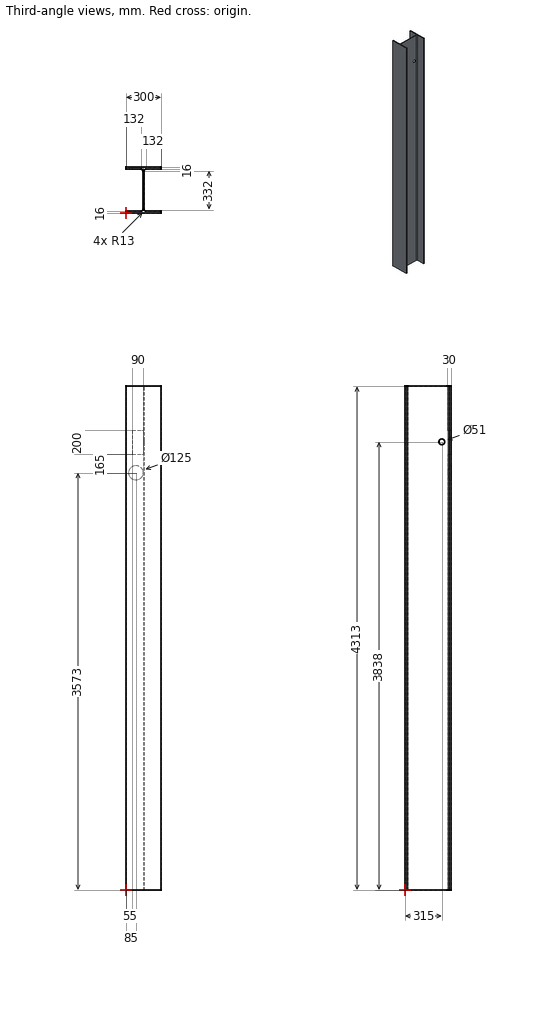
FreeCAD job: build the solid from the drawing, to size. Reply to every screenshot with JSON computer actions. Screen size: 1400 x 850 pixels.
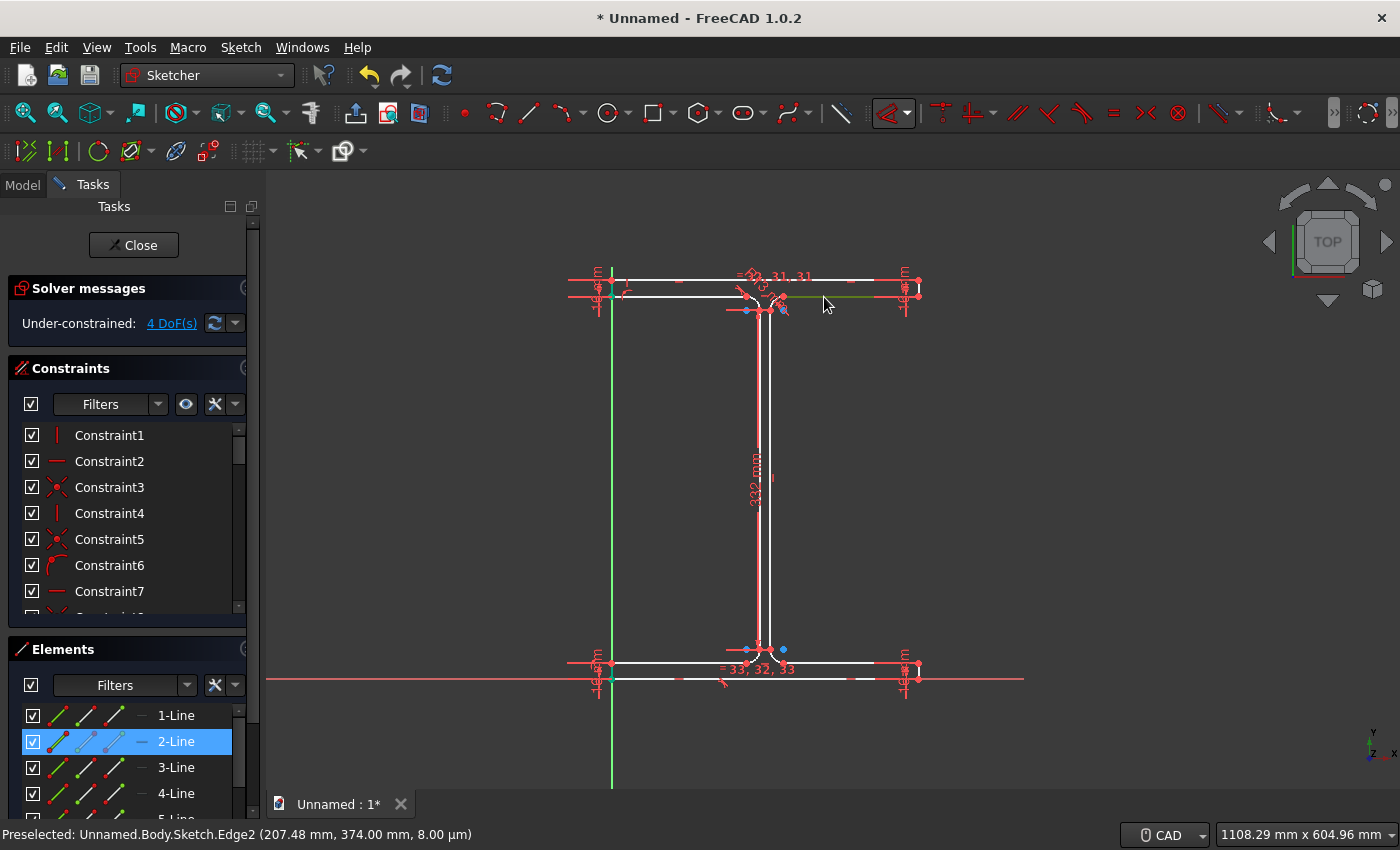
{"action": "left_click", "coordinate": [910, 114]}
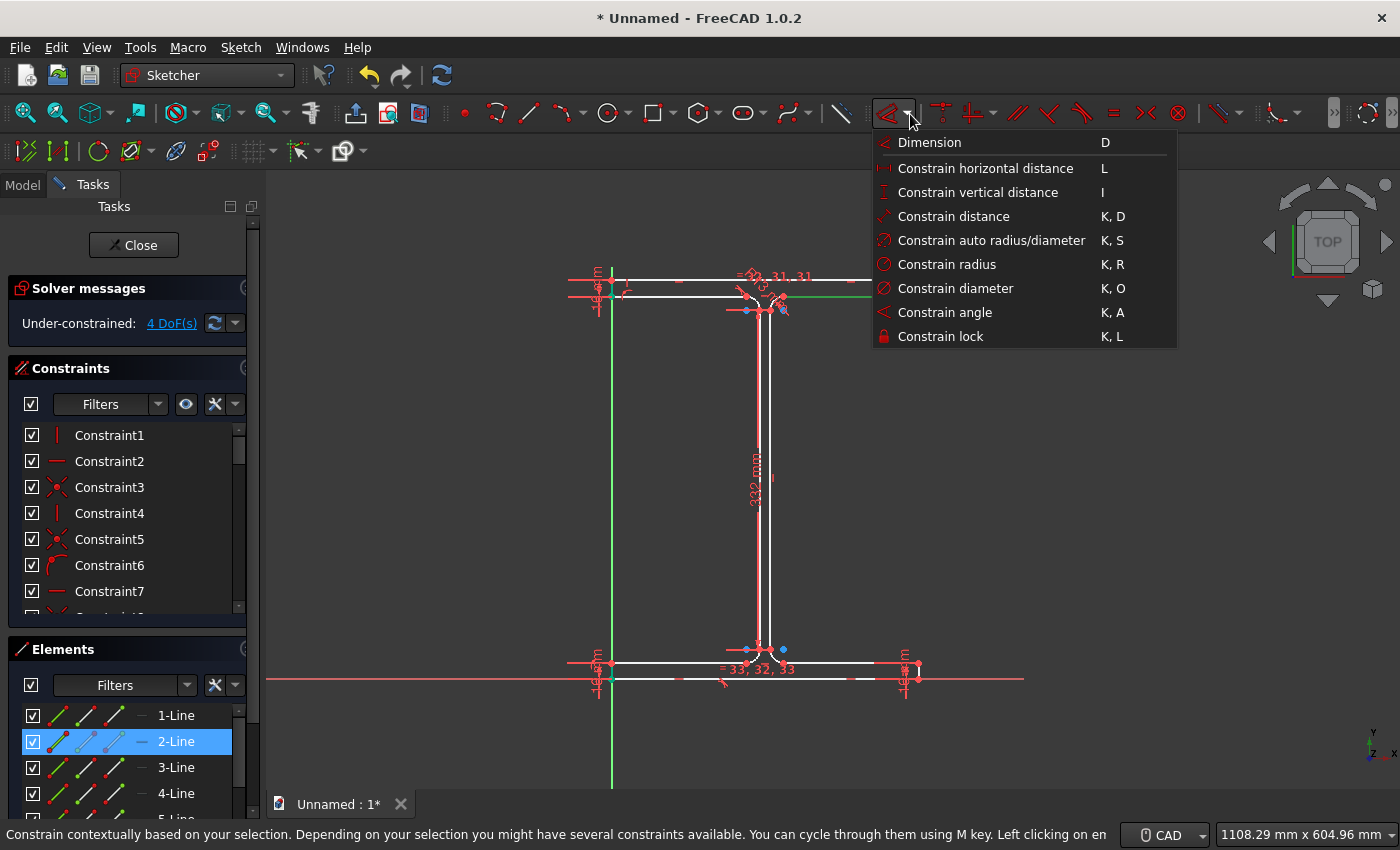
{"action": "left_click", "coordinate": [1025, 168]}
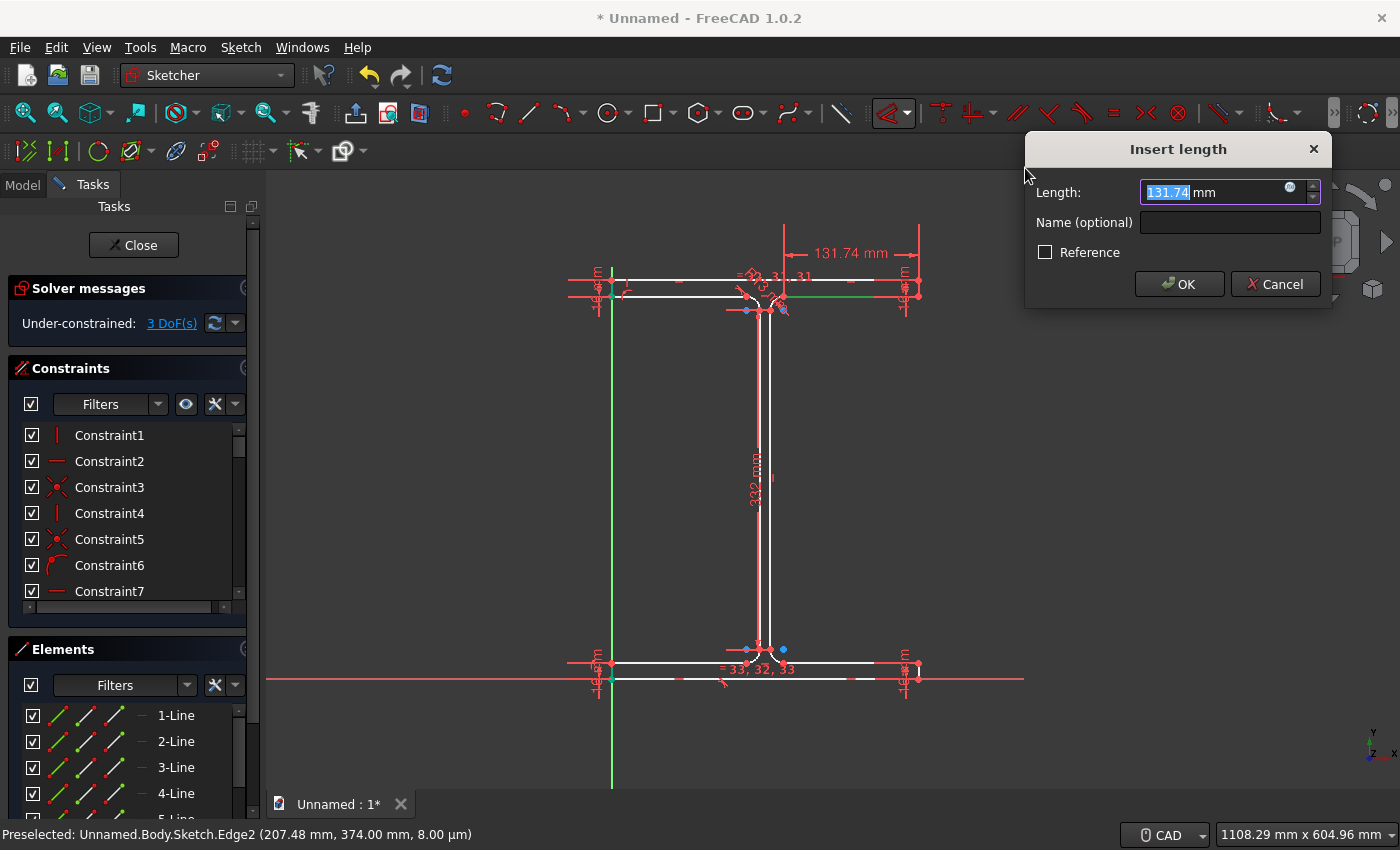
{"action": "type", "text": "132"}
{"action": "key", "text": "Return"}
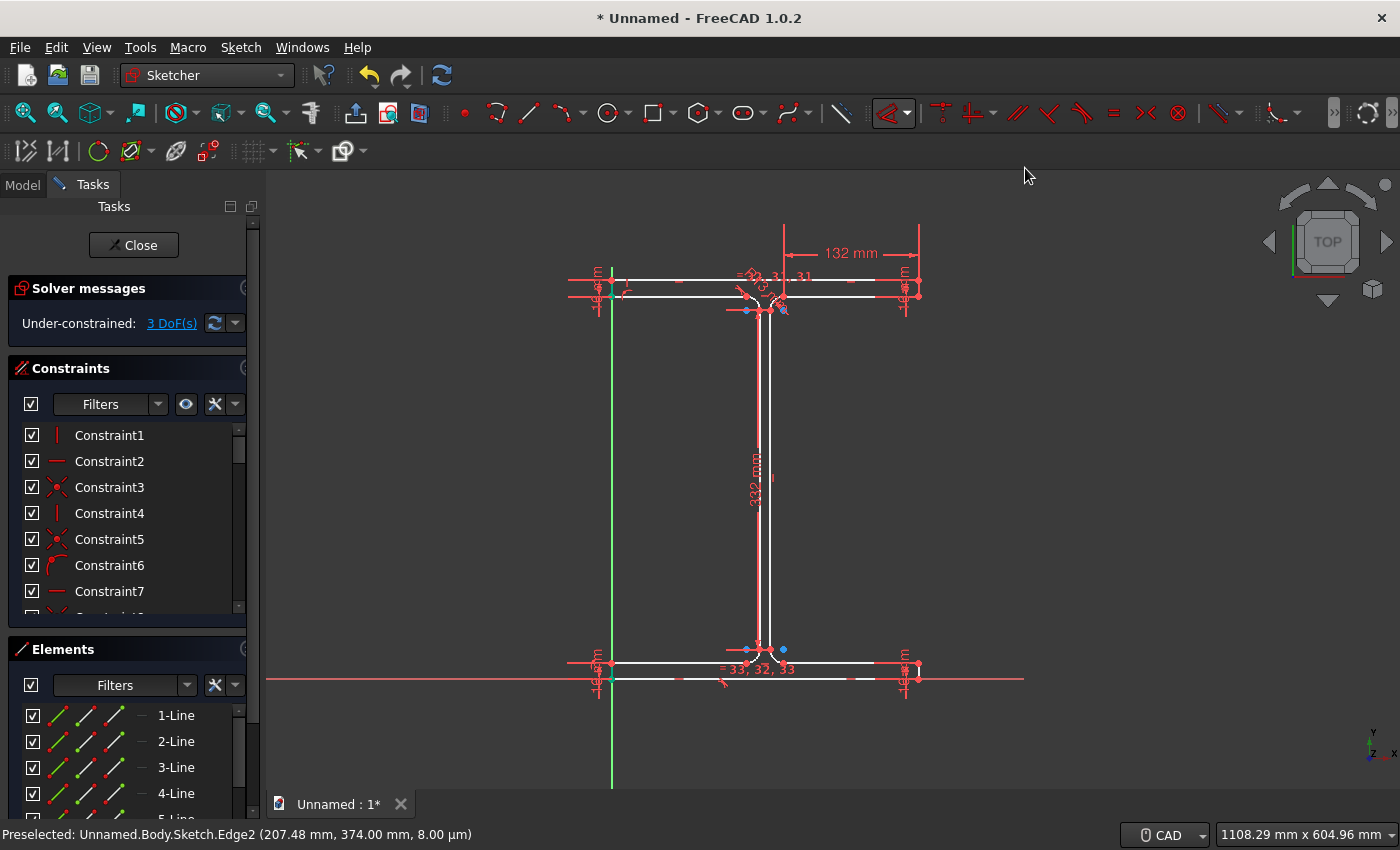
{"action": "left_click", "coordinate": [827, 280]}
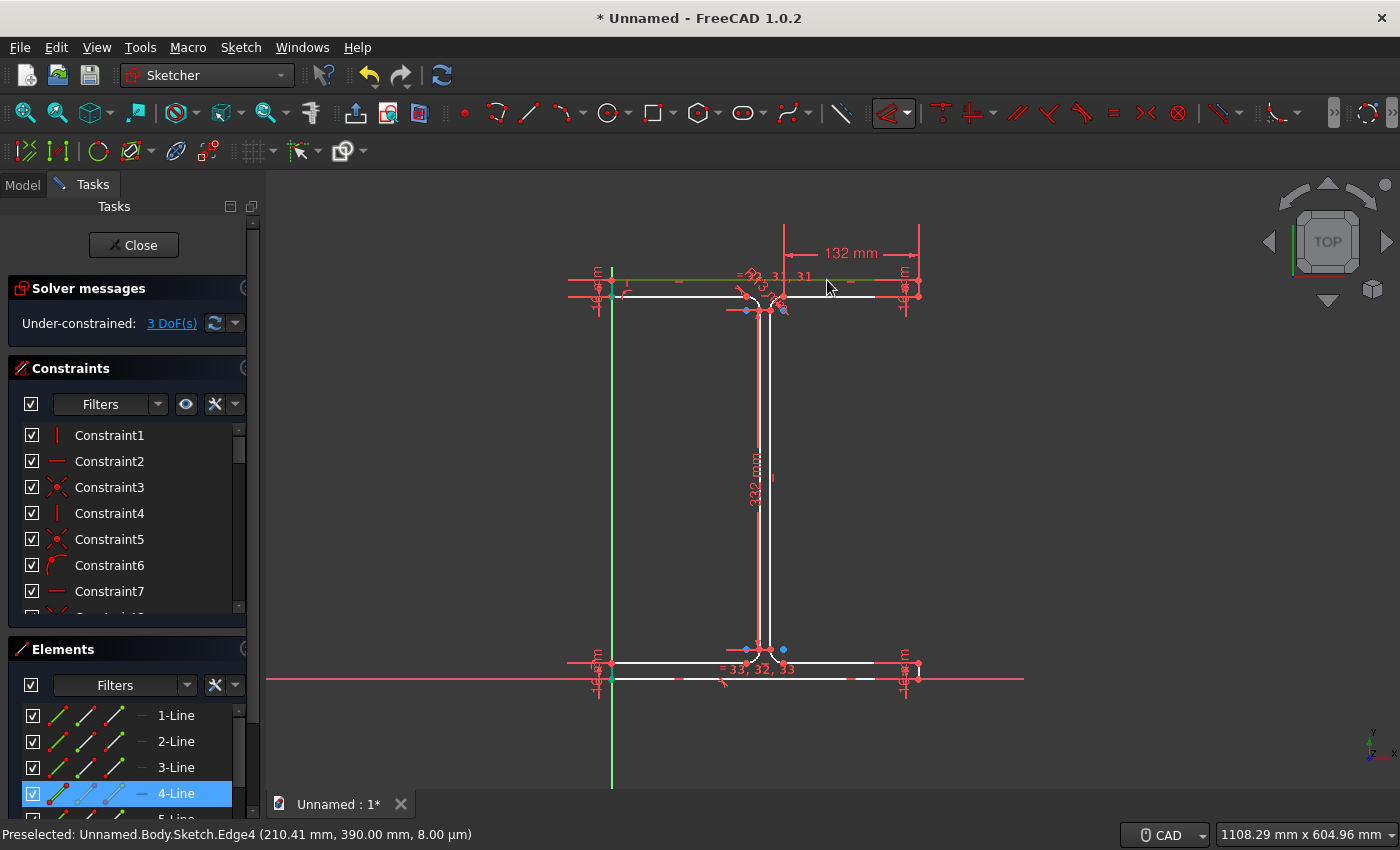
{"action": "key", "text": "l"}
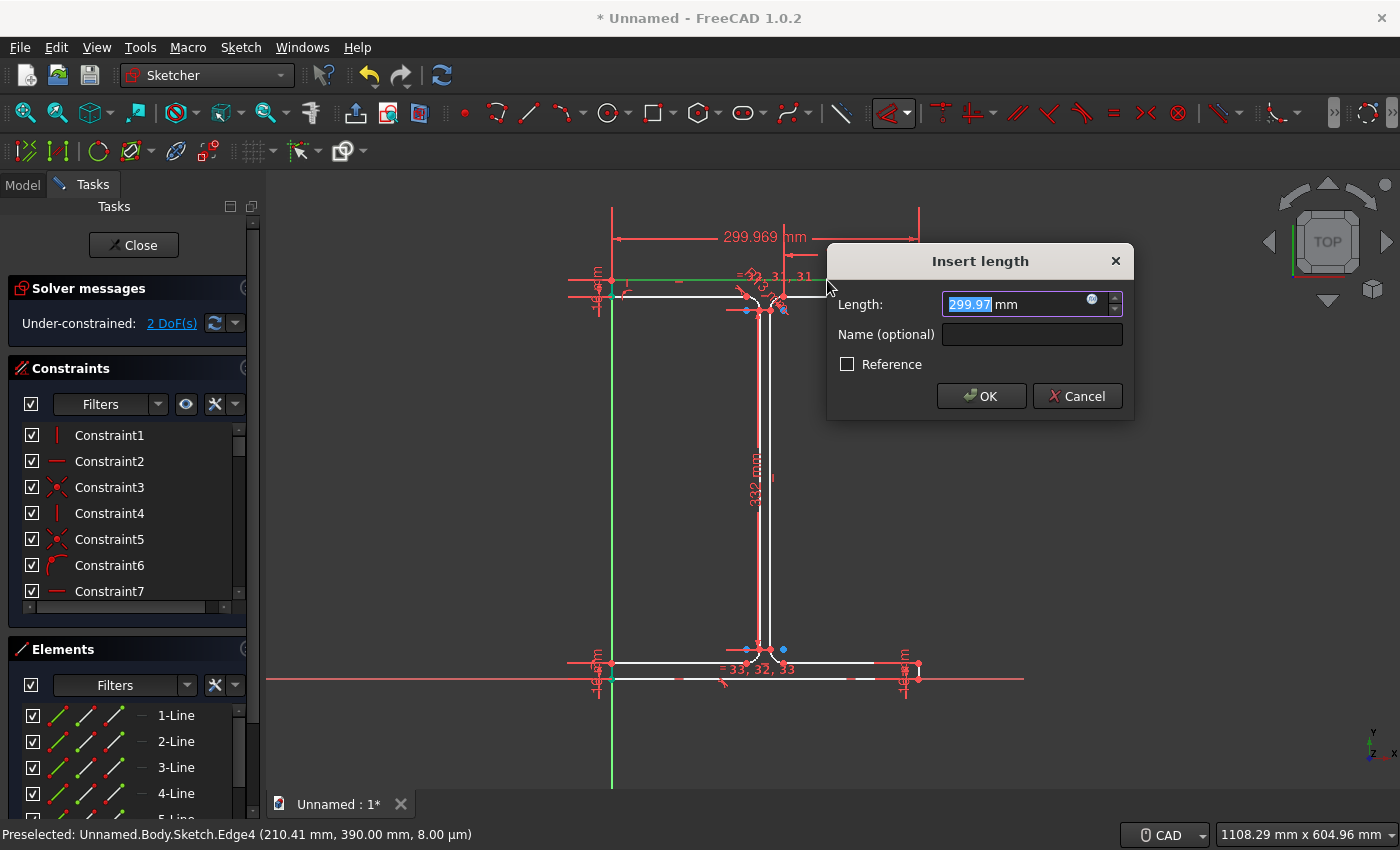
{"action": "type", "text": "300"}
{"action": "key", "text": "Return"}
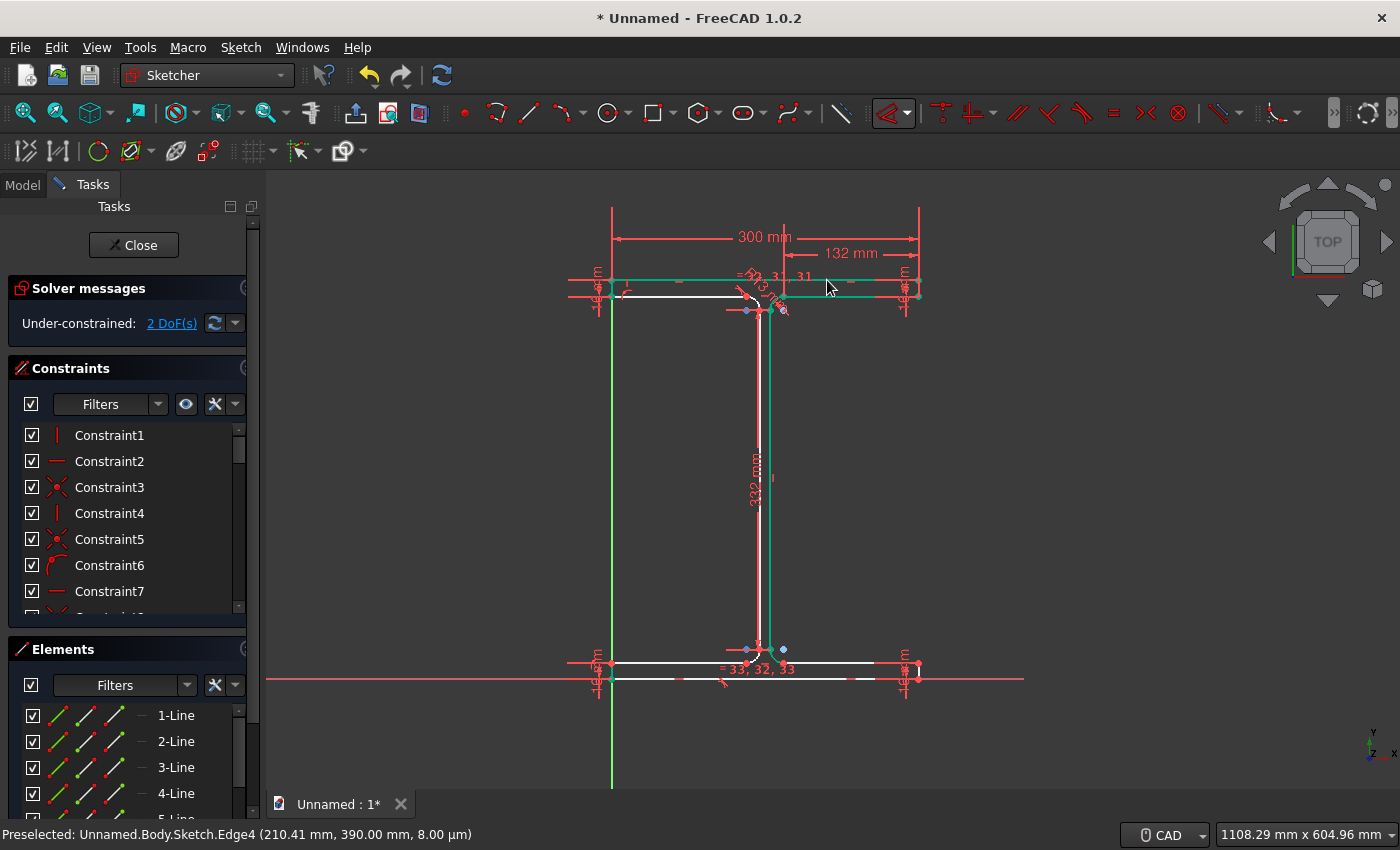
{"action": "left_click", "coordinate": [652, 297]}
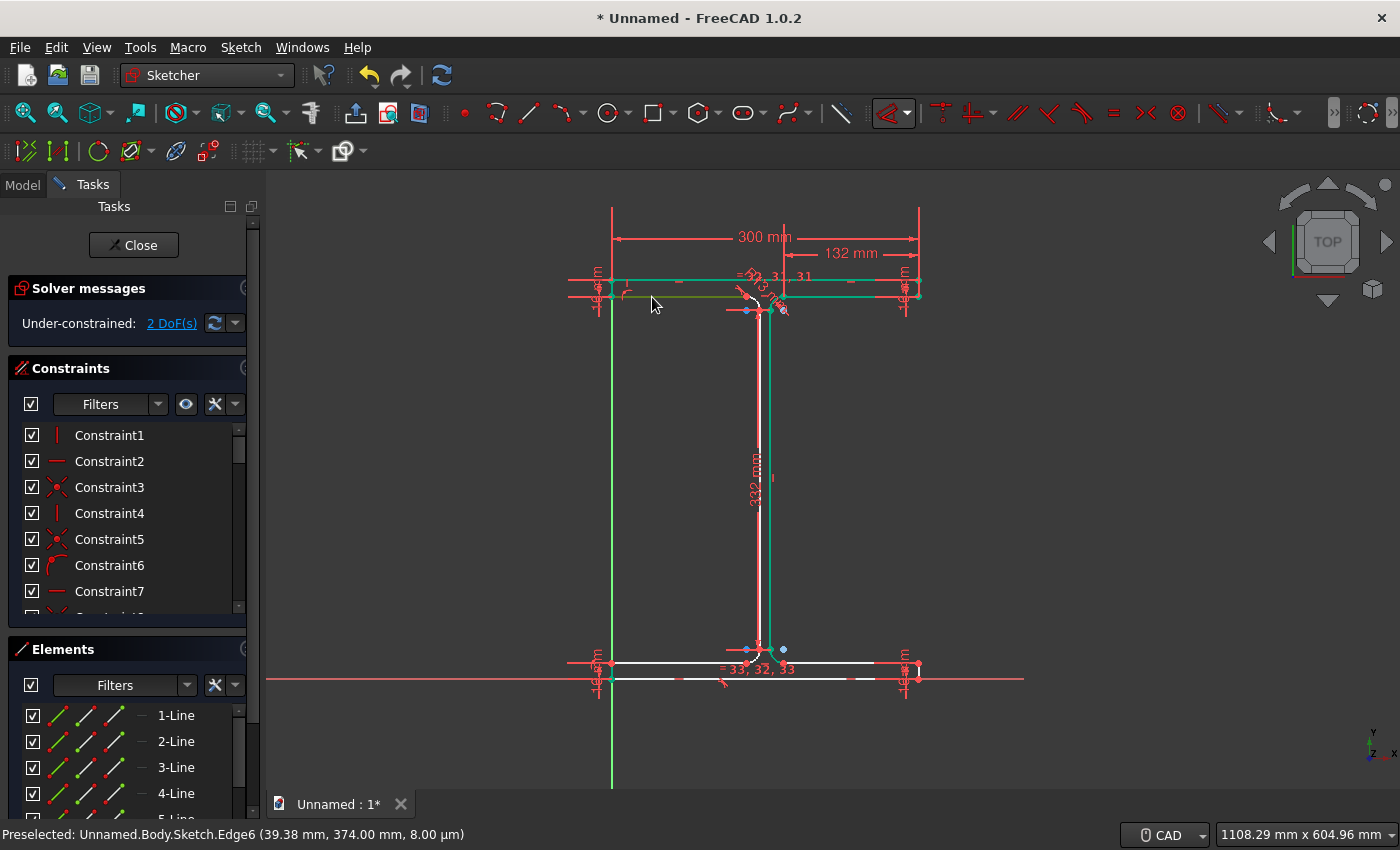
{"action": "key", "text": "l"}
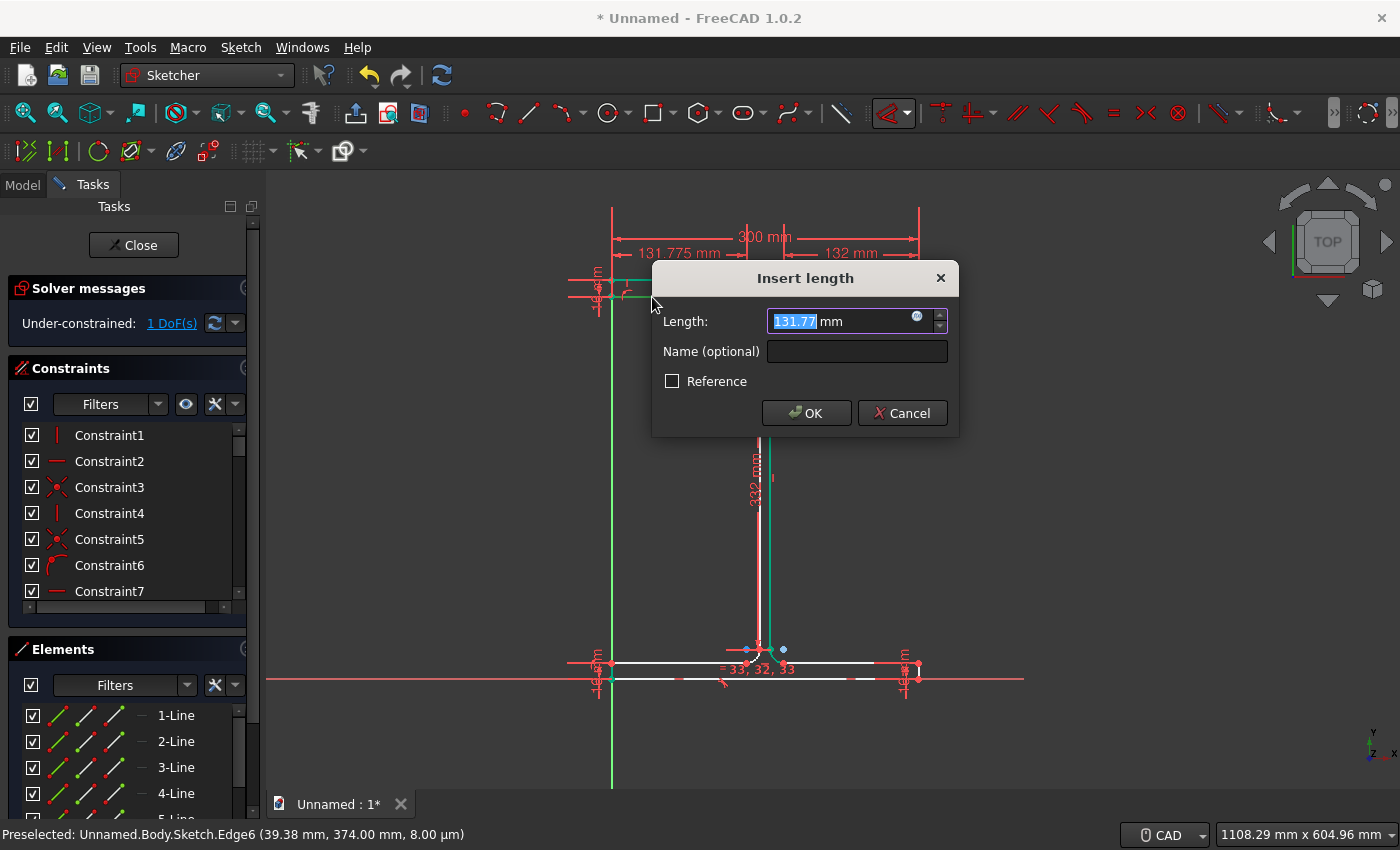
{"action": "type", "text": "132"}
{"action": "key", "text": "Return"}